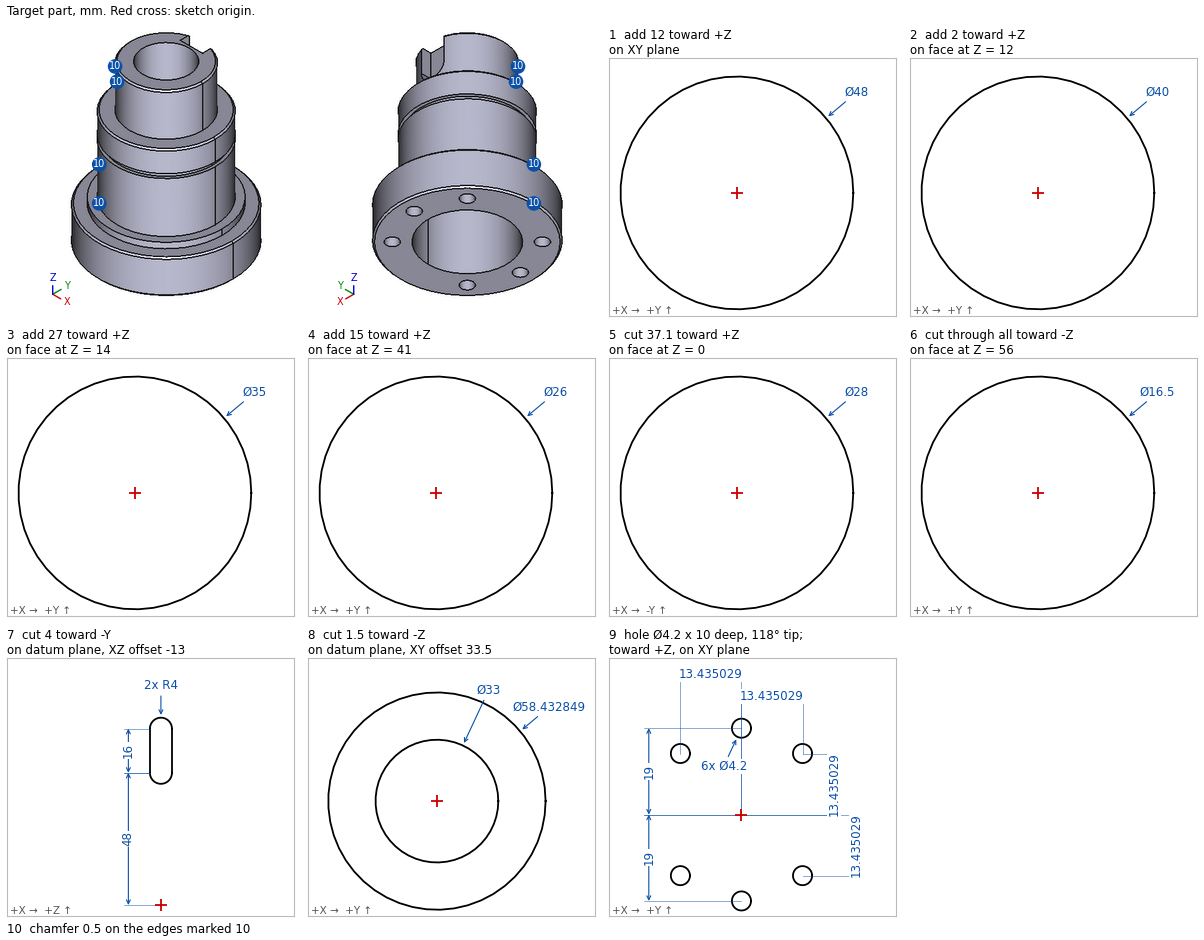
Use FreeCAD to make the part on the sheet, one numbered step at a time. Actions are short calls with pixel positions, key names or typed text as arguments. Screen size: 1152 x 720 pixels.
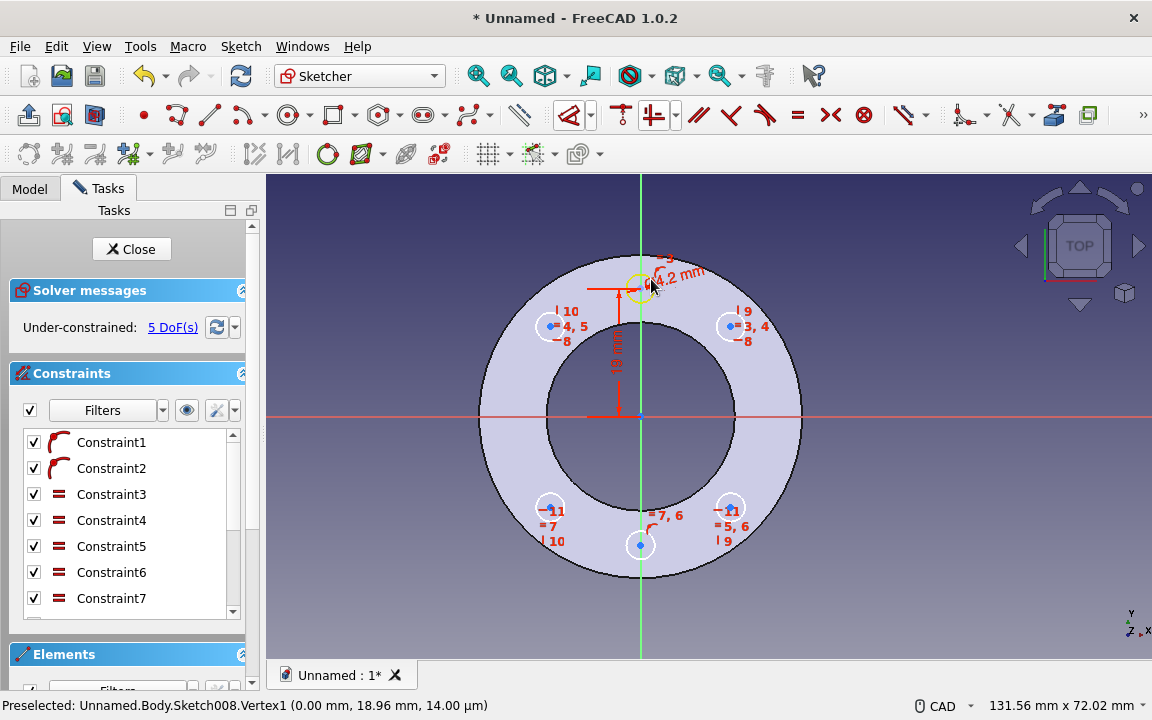
click(641, 545)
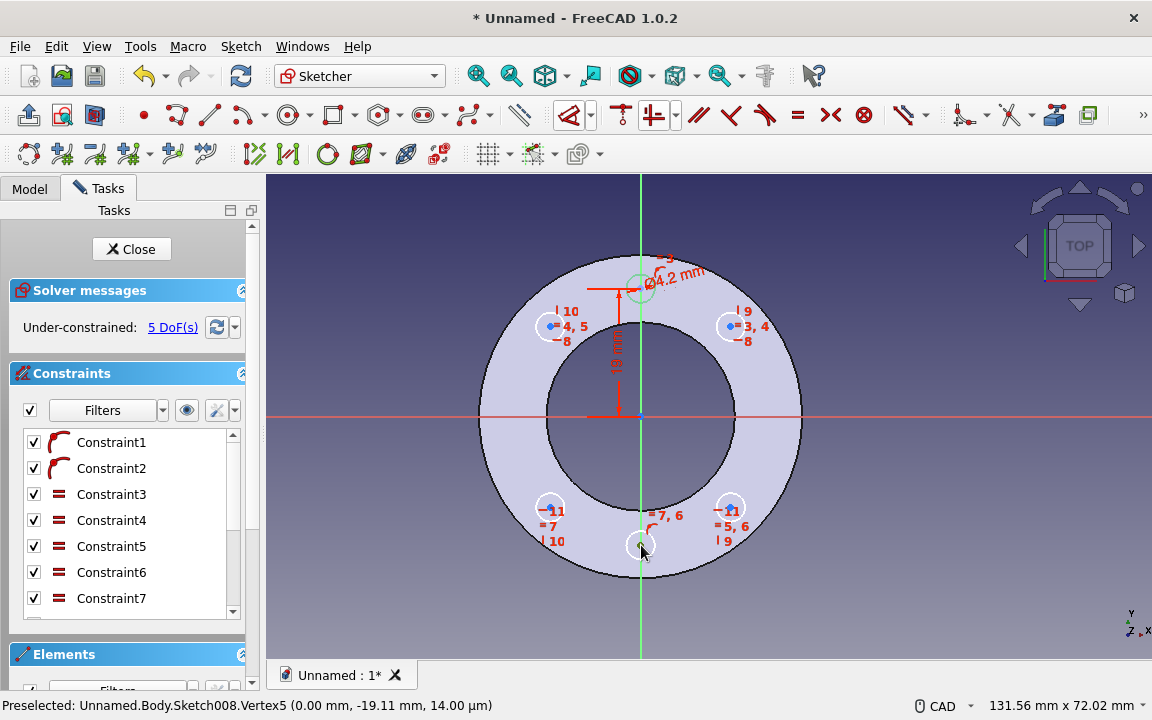
key(i)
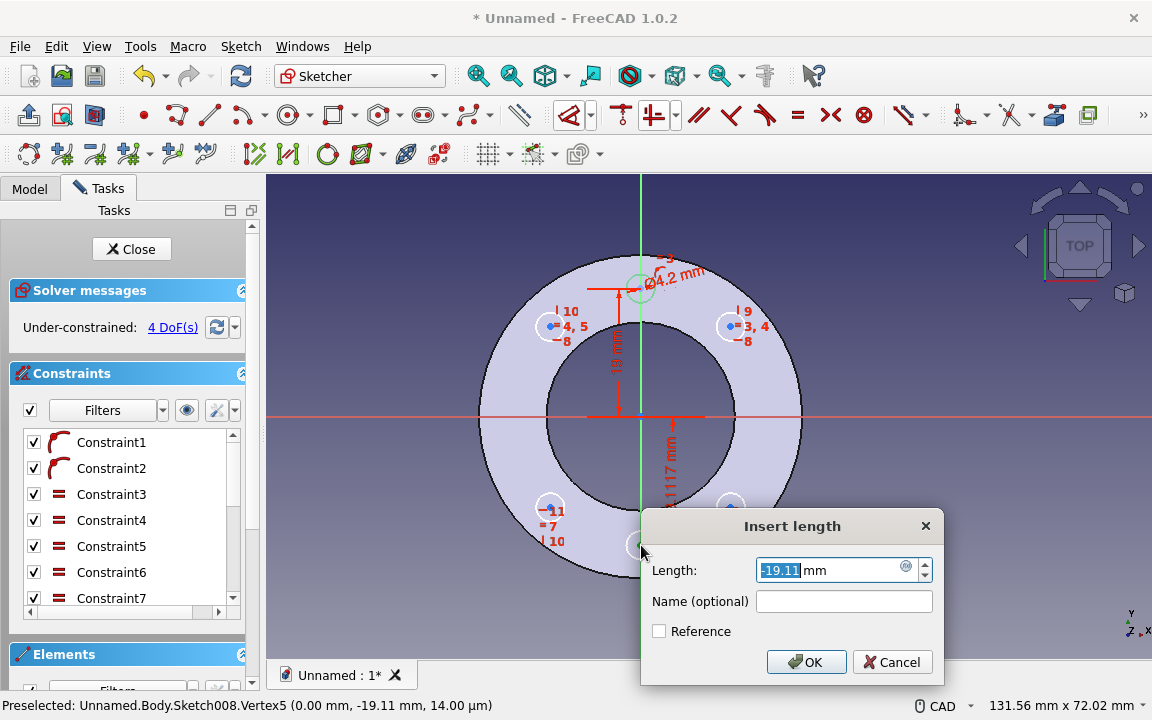
text(-19)
key(Return)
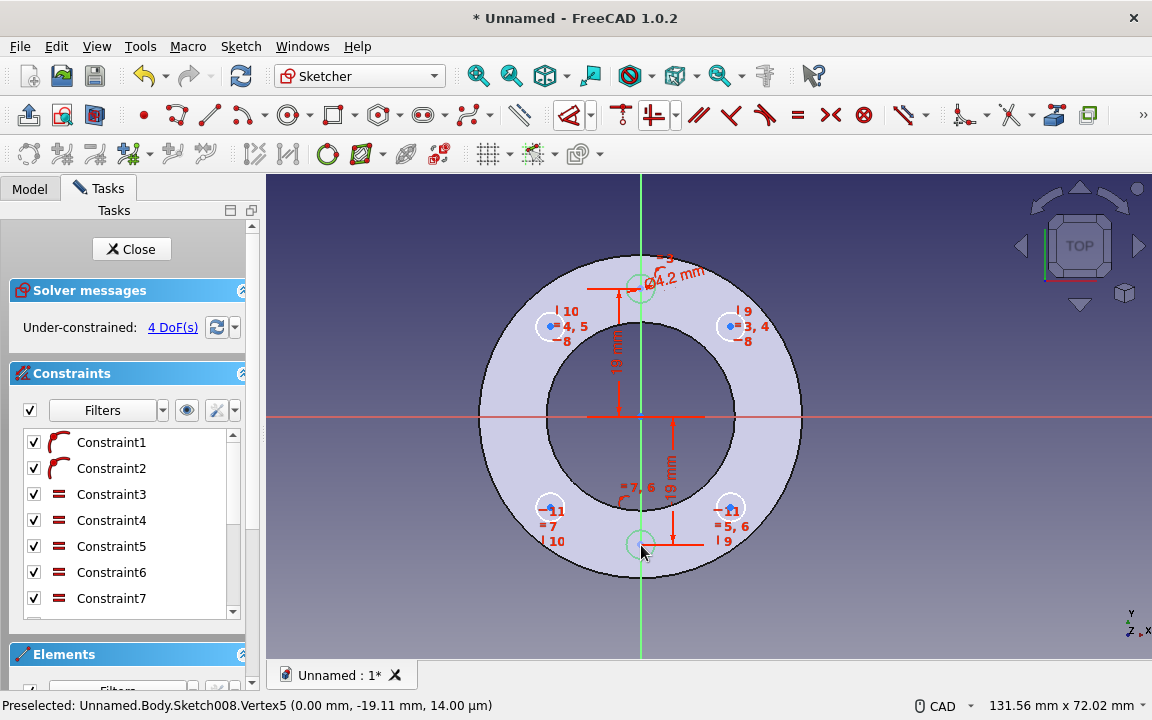
click(731, 327)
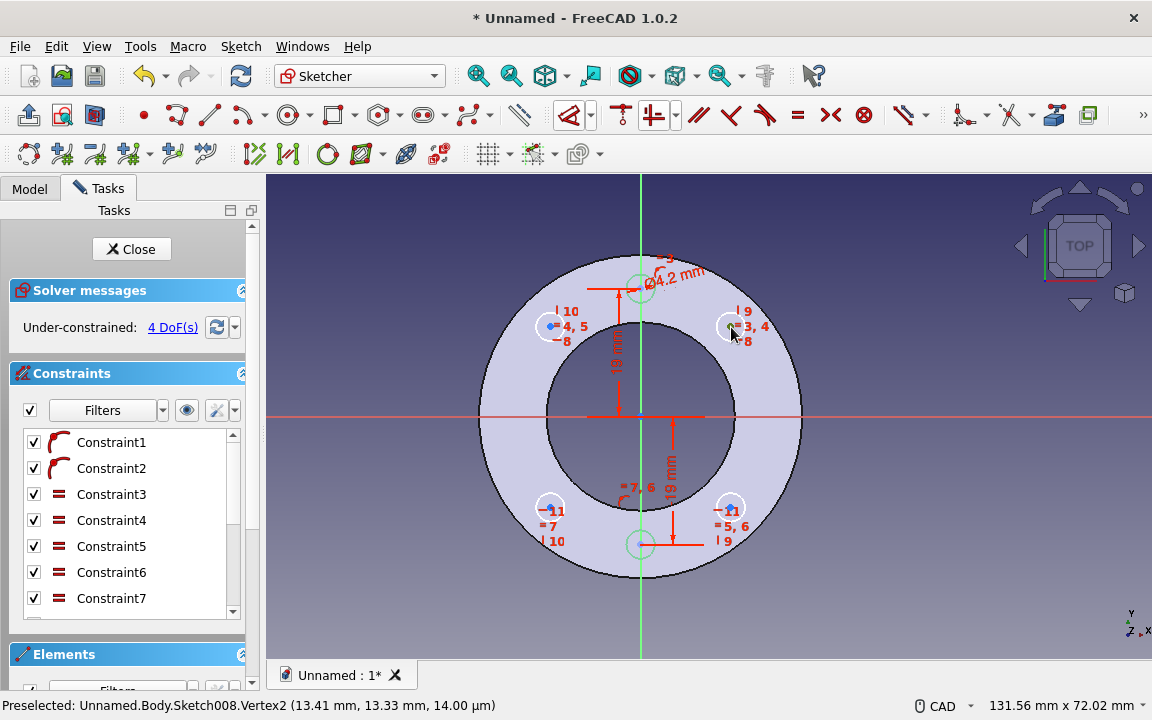
key(l)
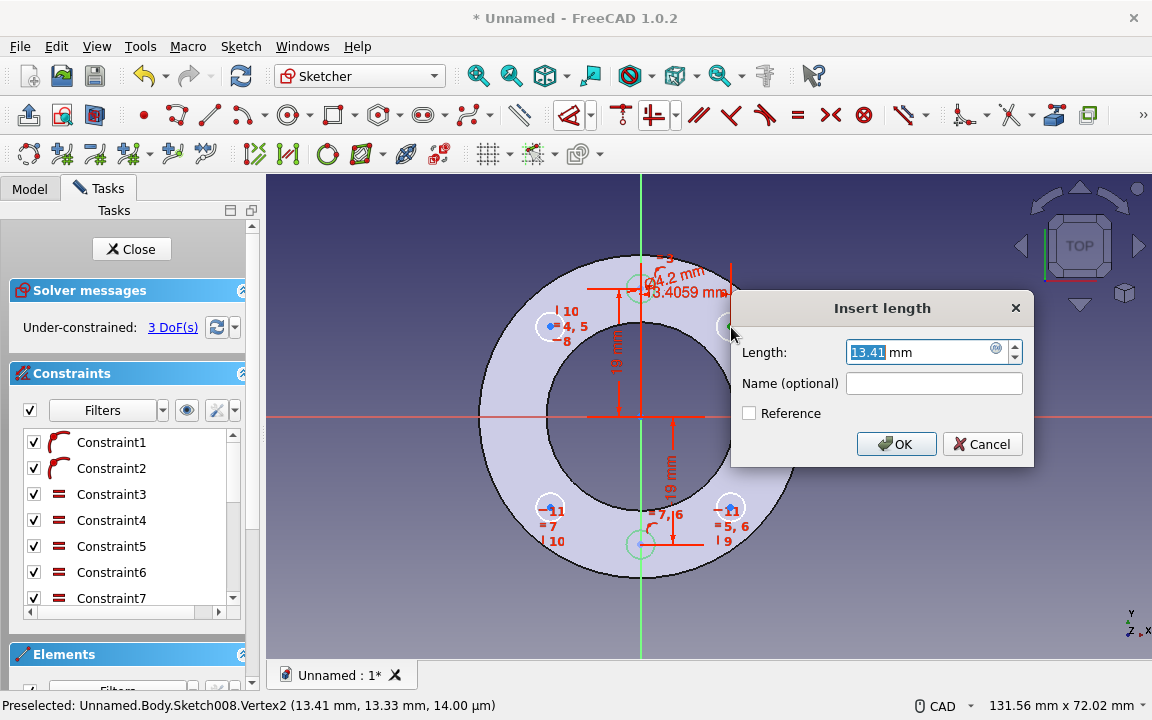
text(13.435029)
key(Return)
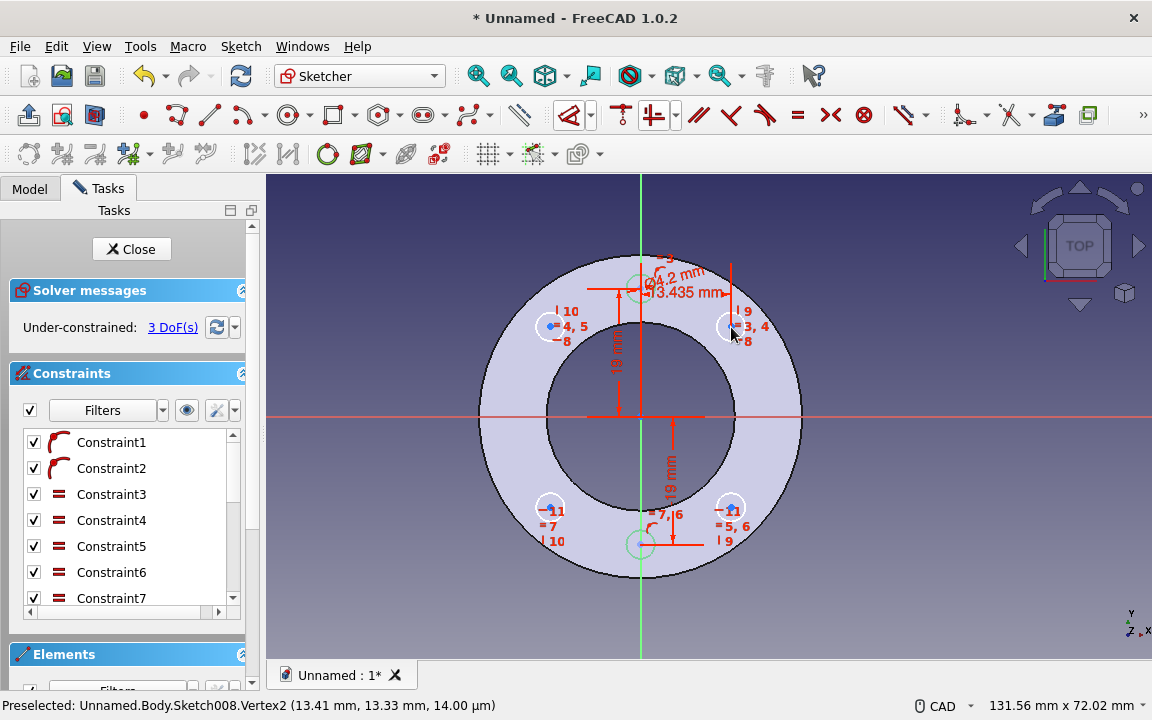
click(731, 327)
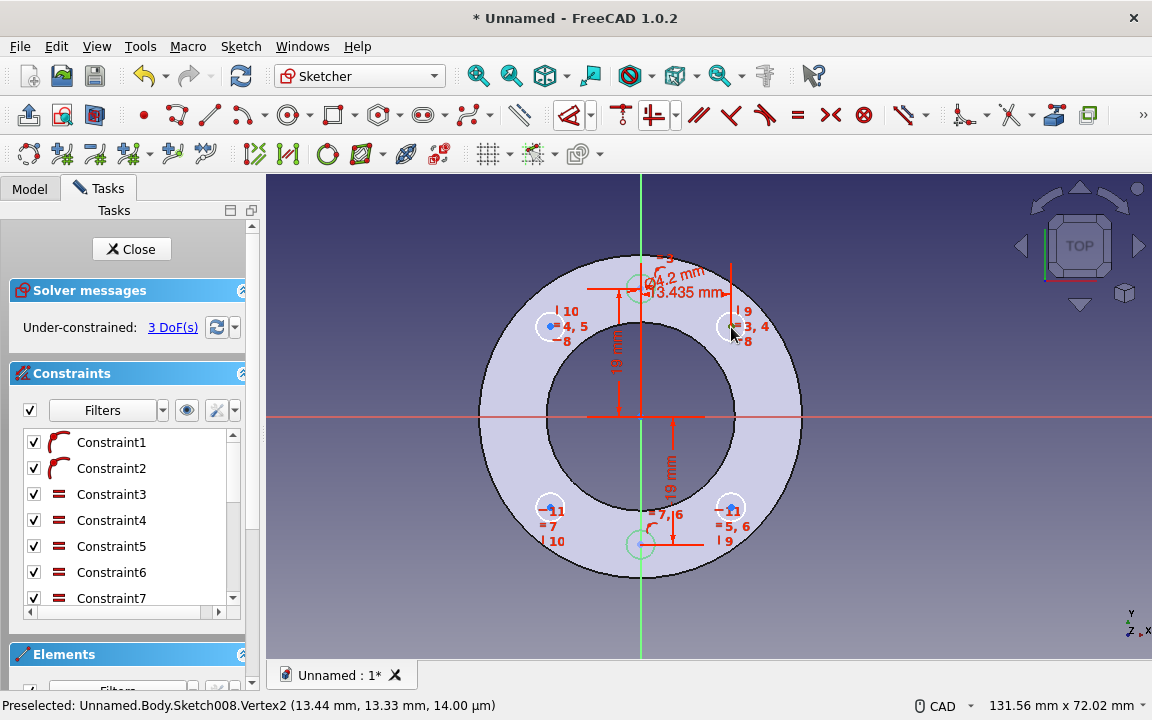
key(i)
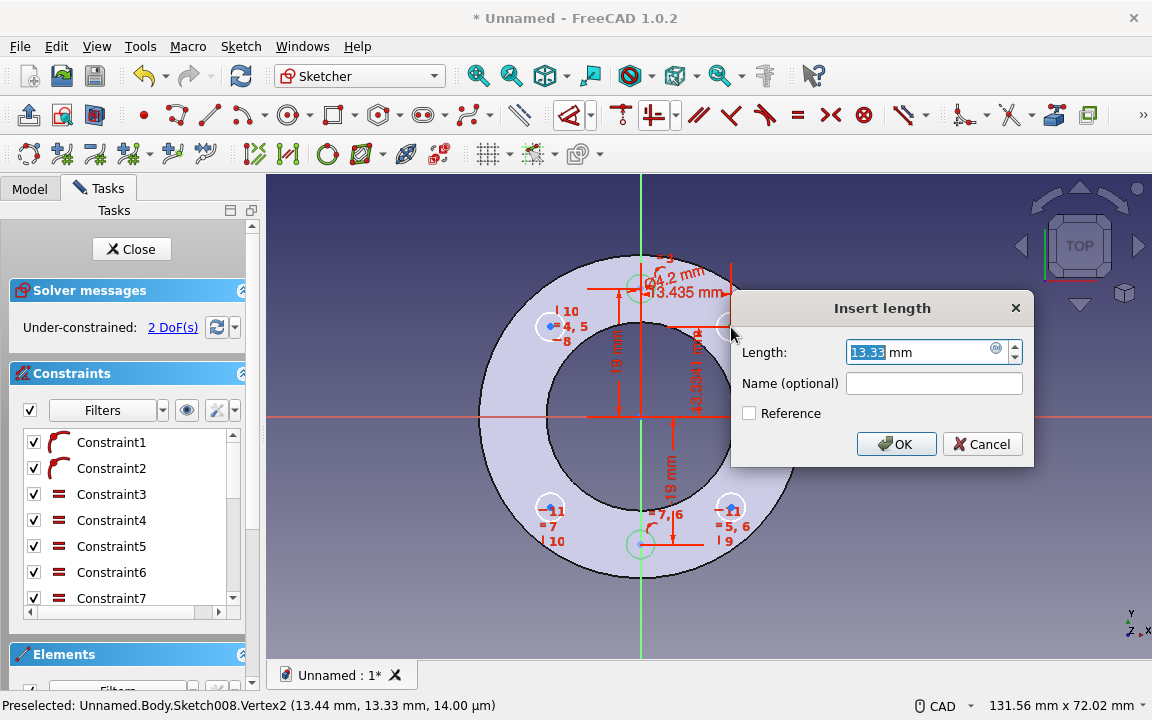
text(13.435029)
key(Return)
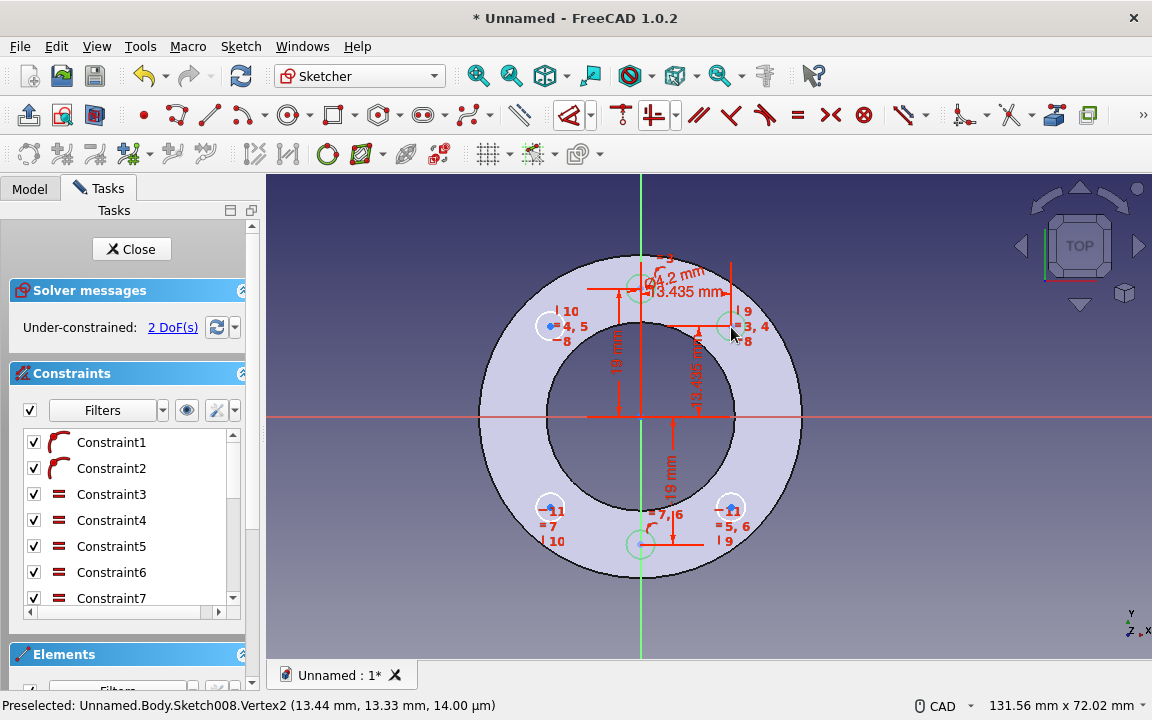
click(550, 326)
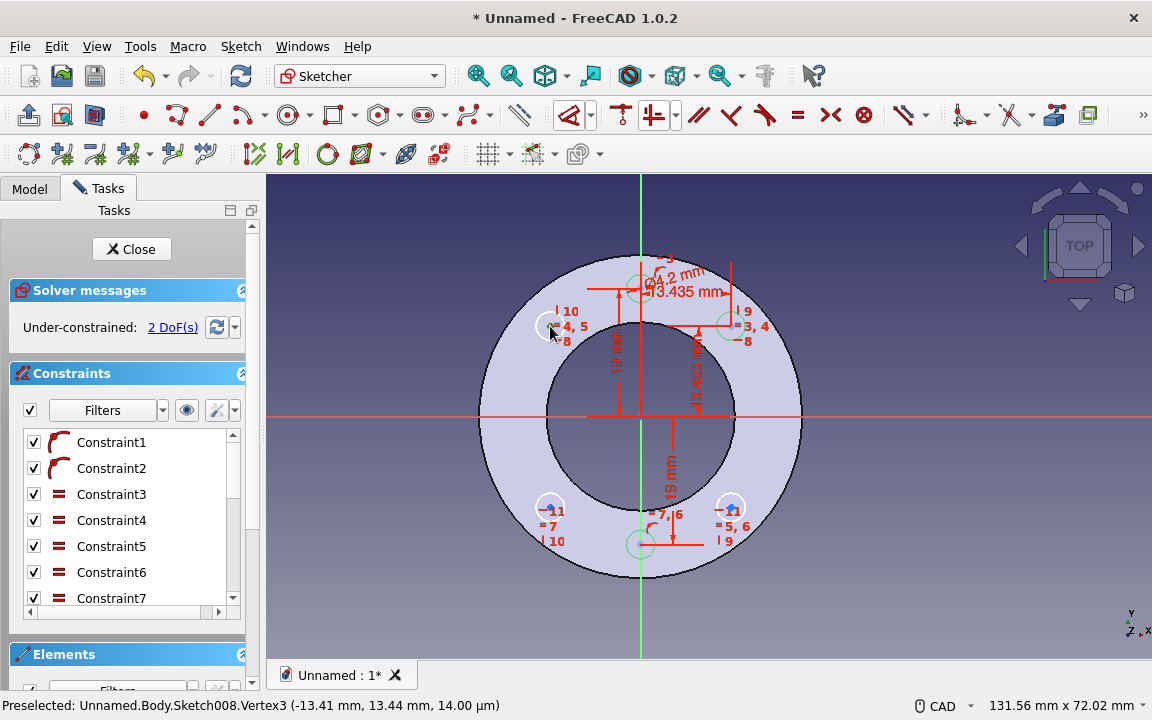
key(l)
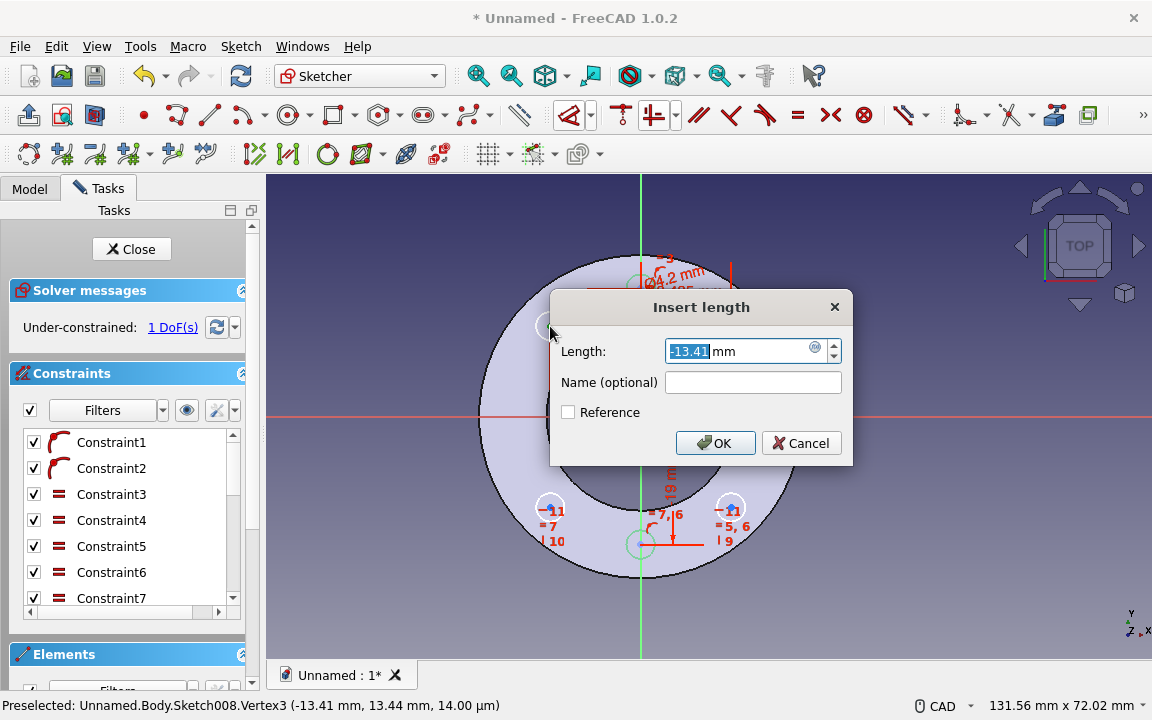
text(-13.435029)
key(Return)